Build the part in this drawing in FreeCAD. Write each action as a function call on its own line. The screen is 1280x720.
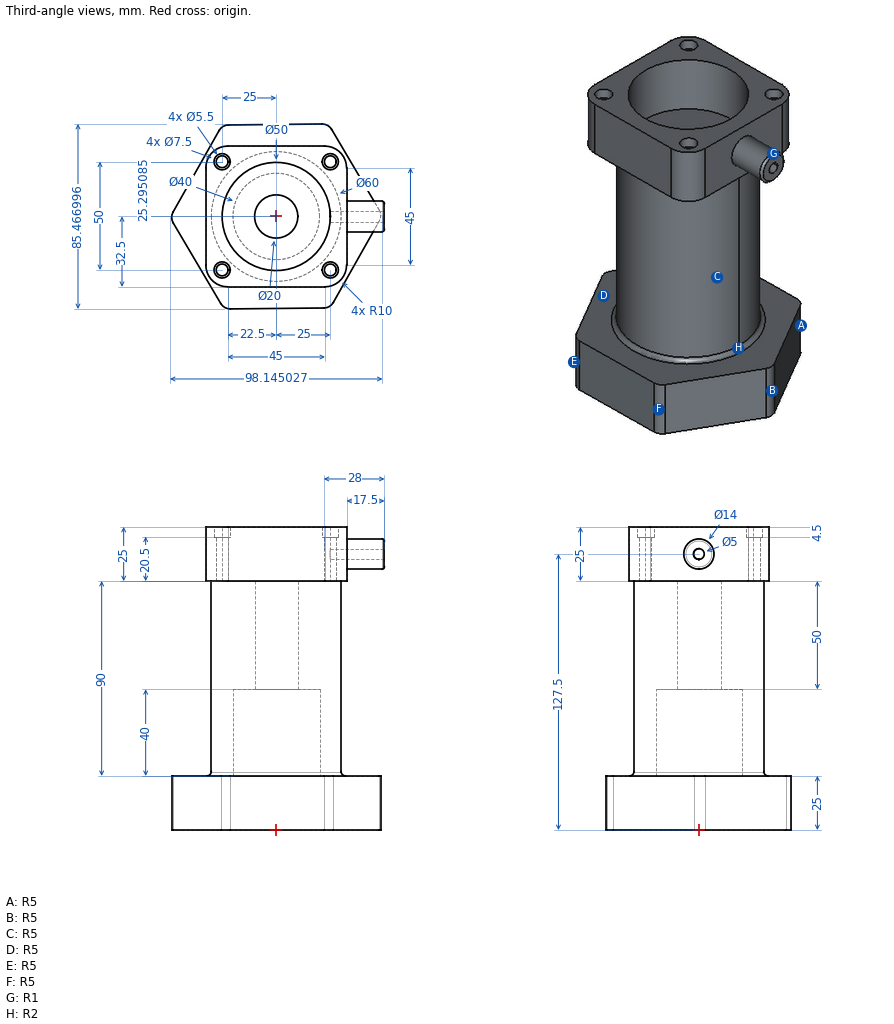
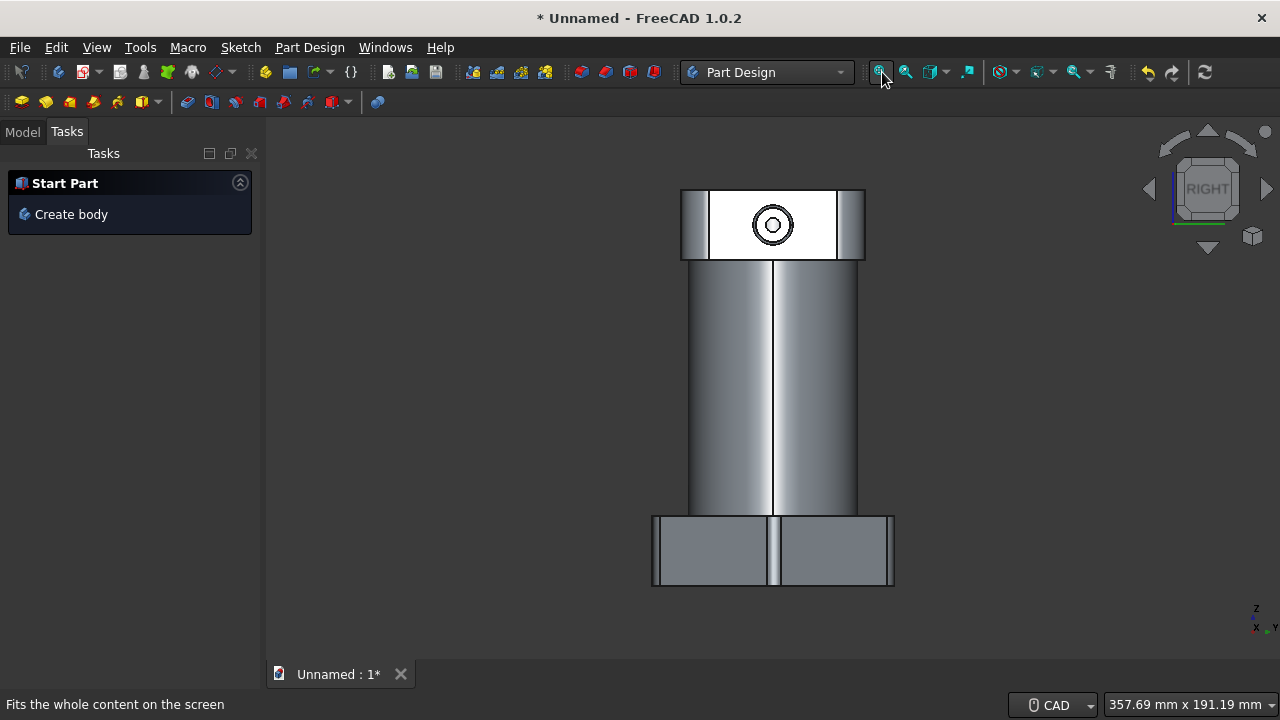
key(5)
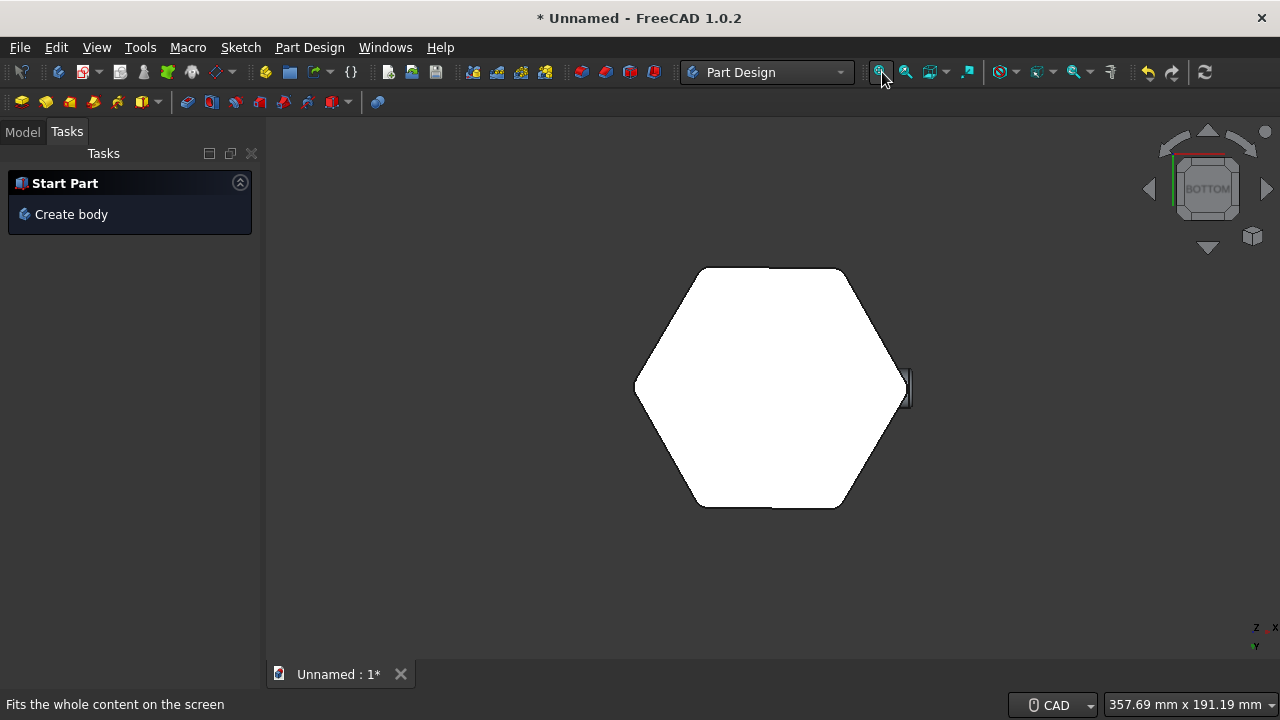
click(882, 72)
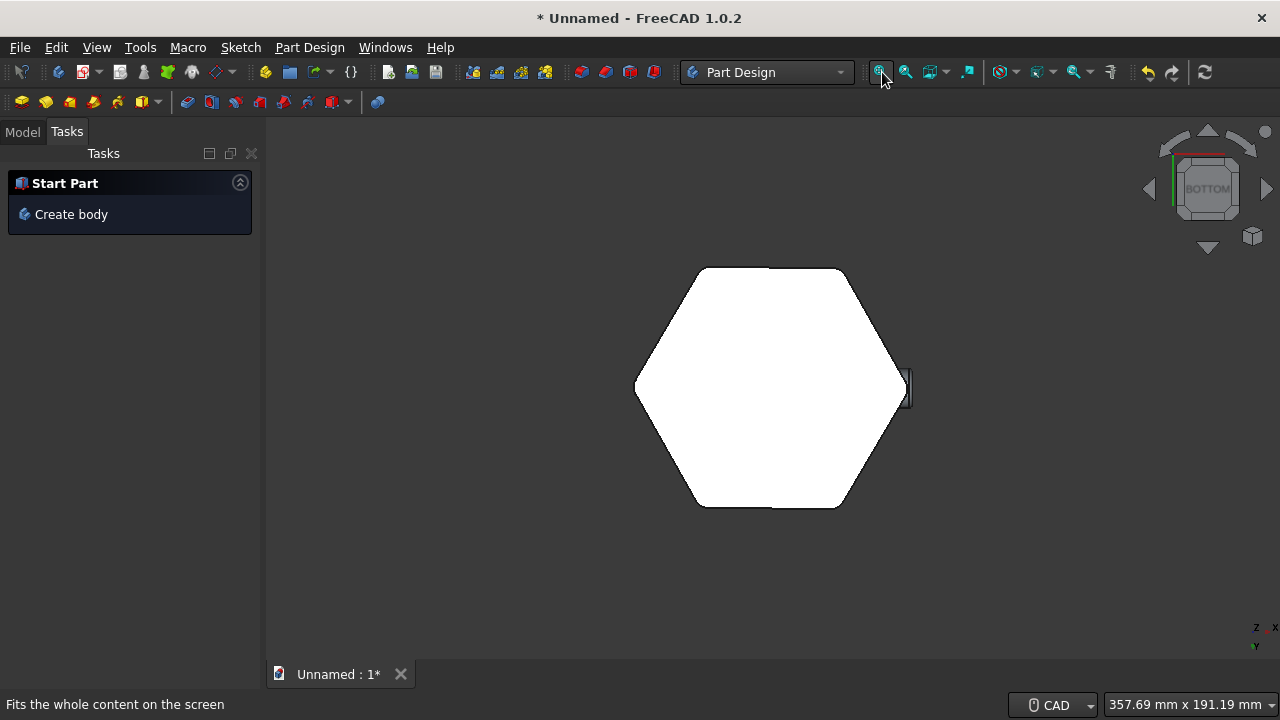
key(4)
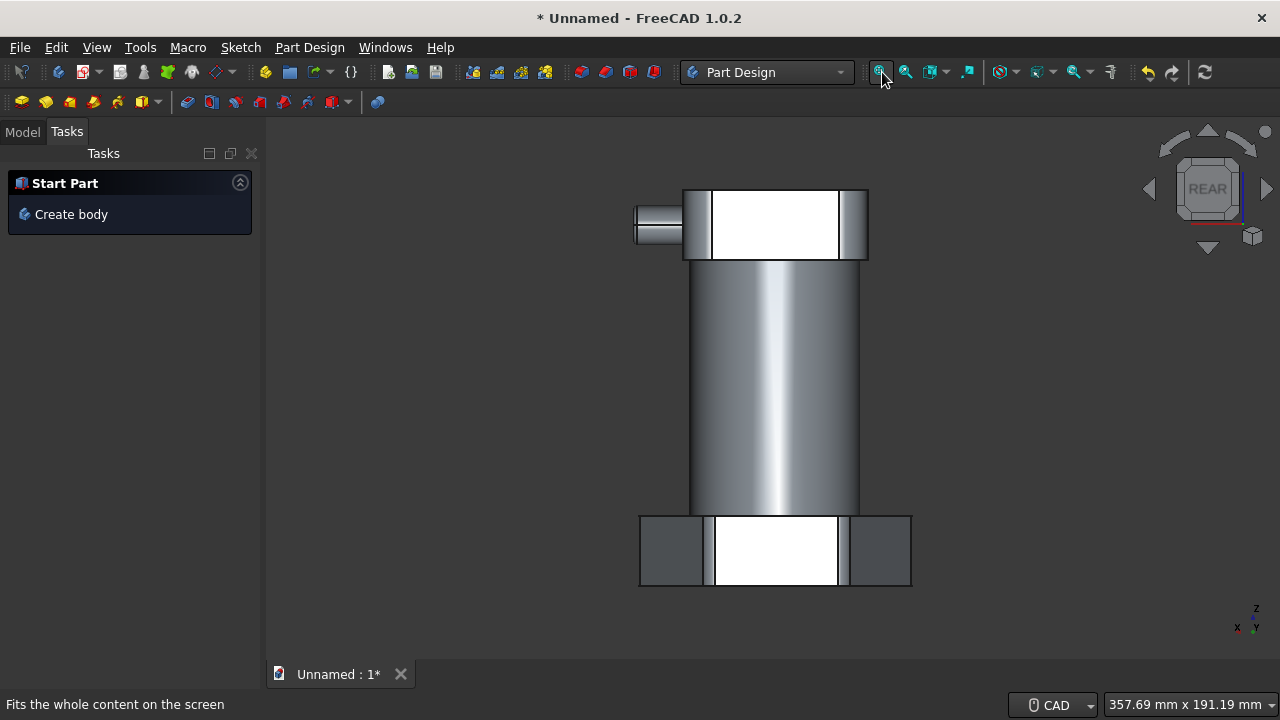
key(6)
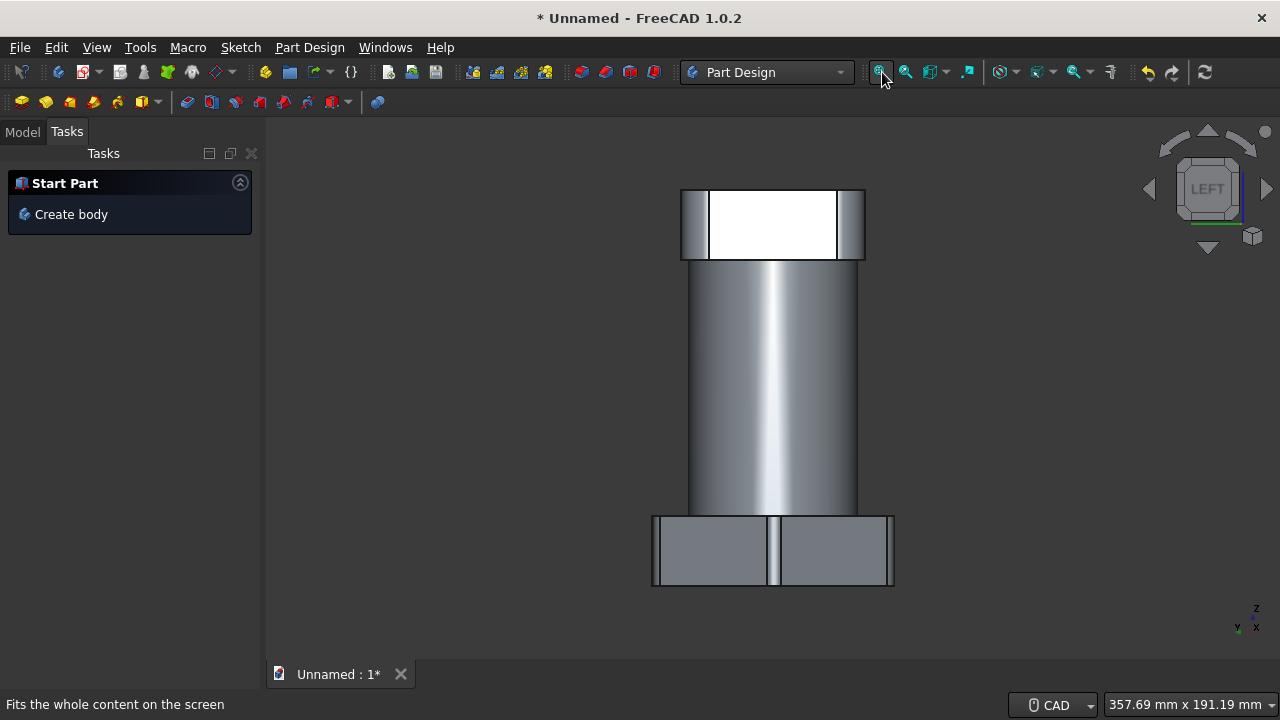
key(v)
key(3)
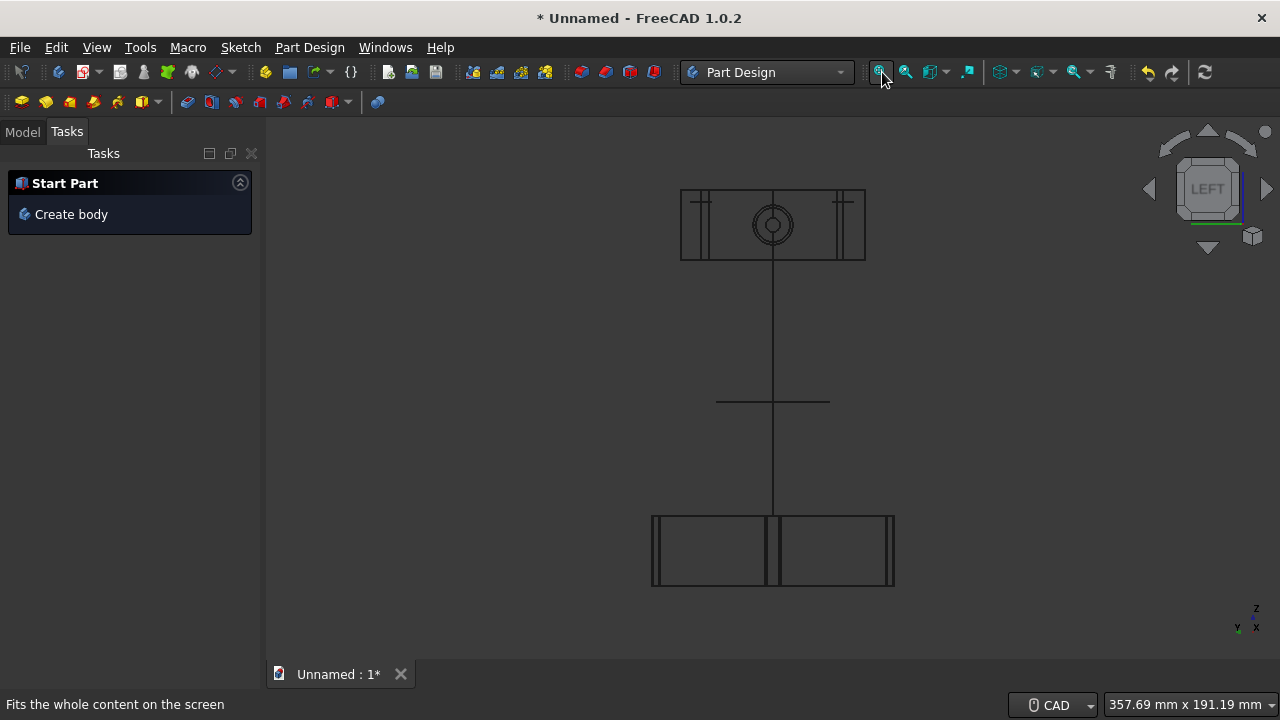
key(0)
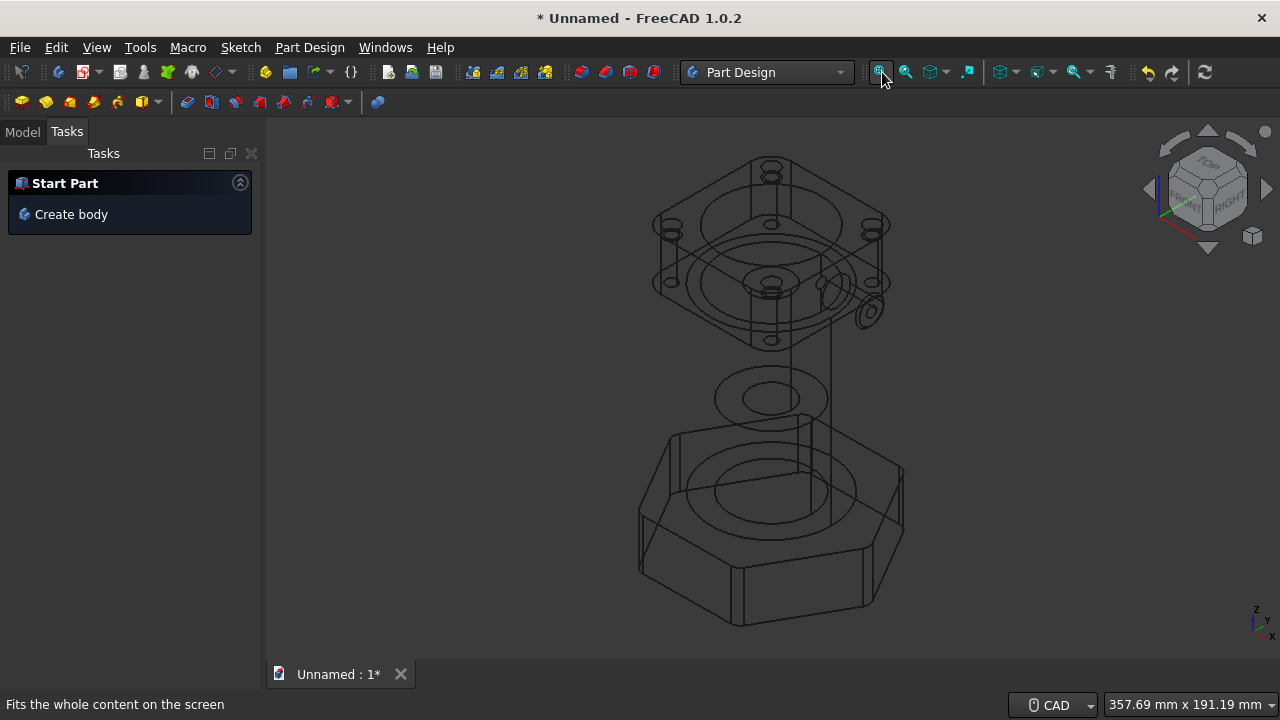
click(711, 455)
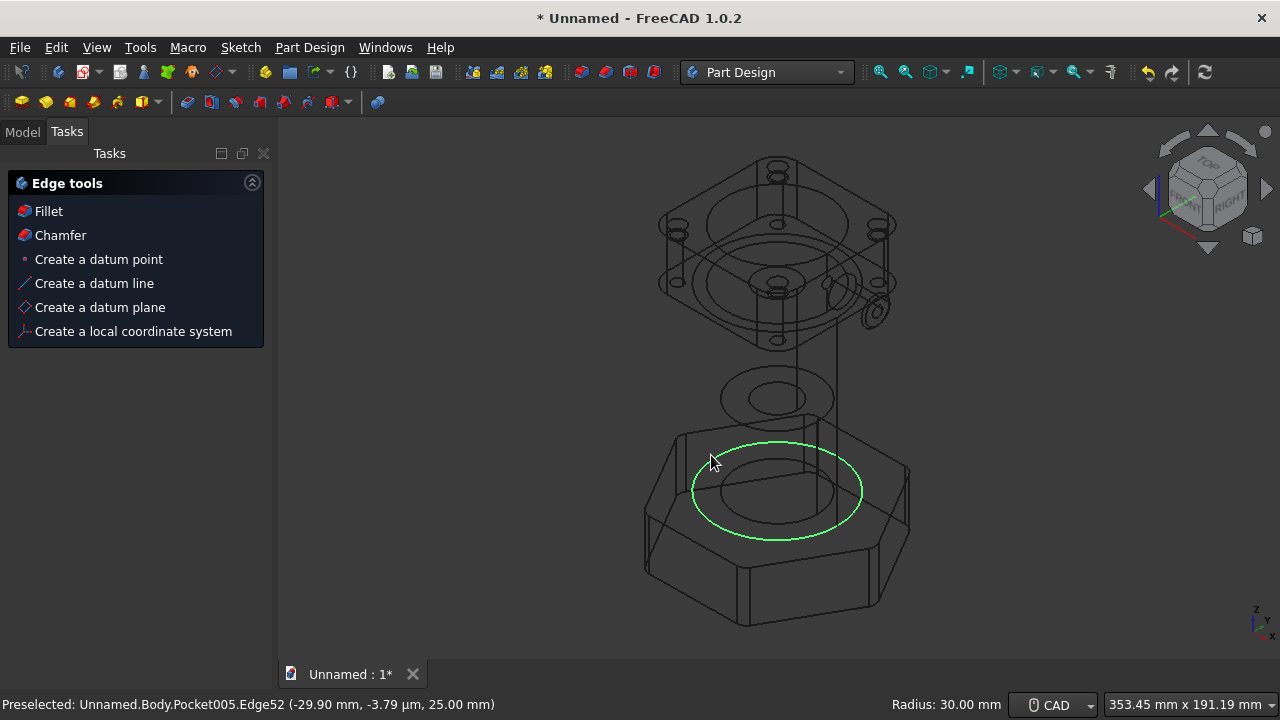
key(v)
key(1)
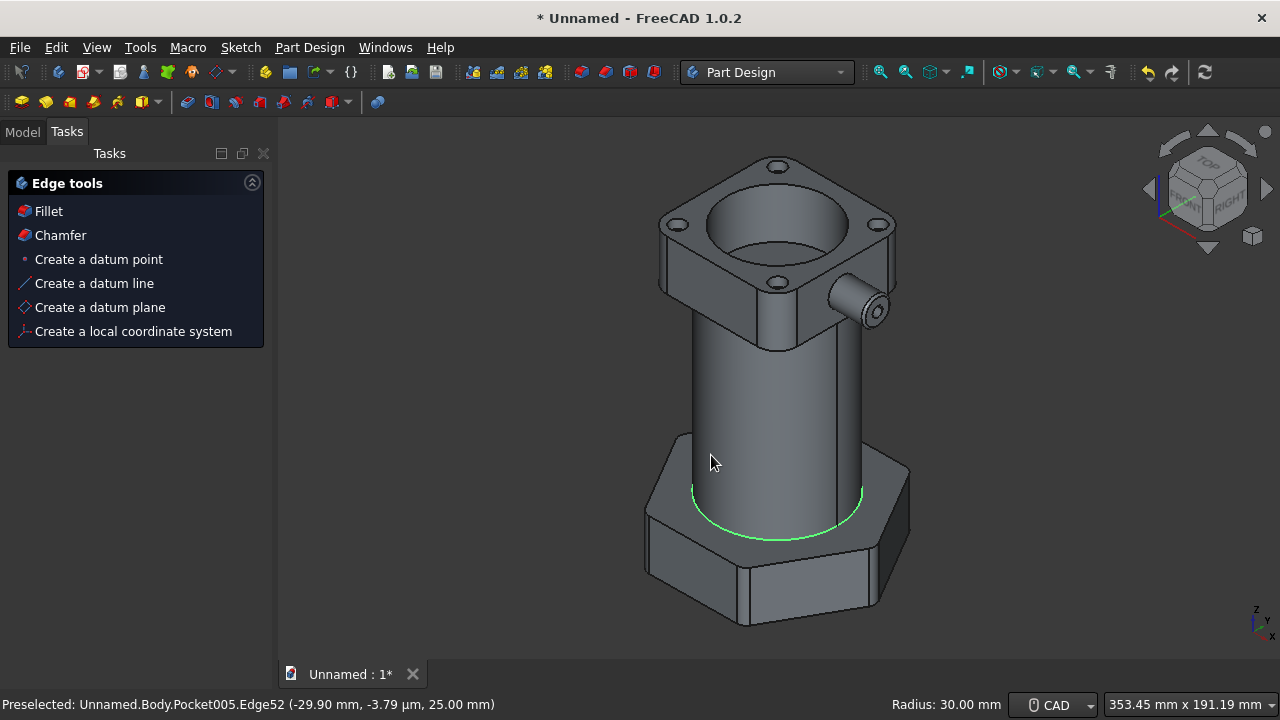
click(582, 72)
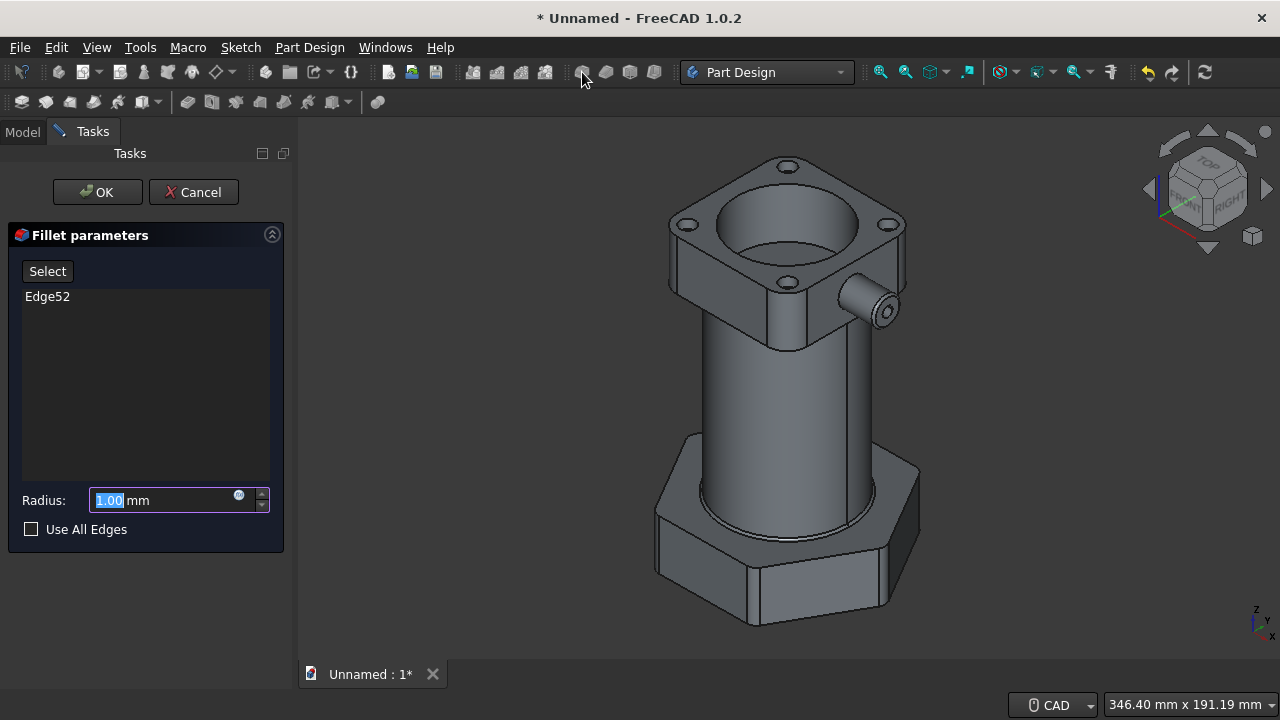
text(2)
key(Tab)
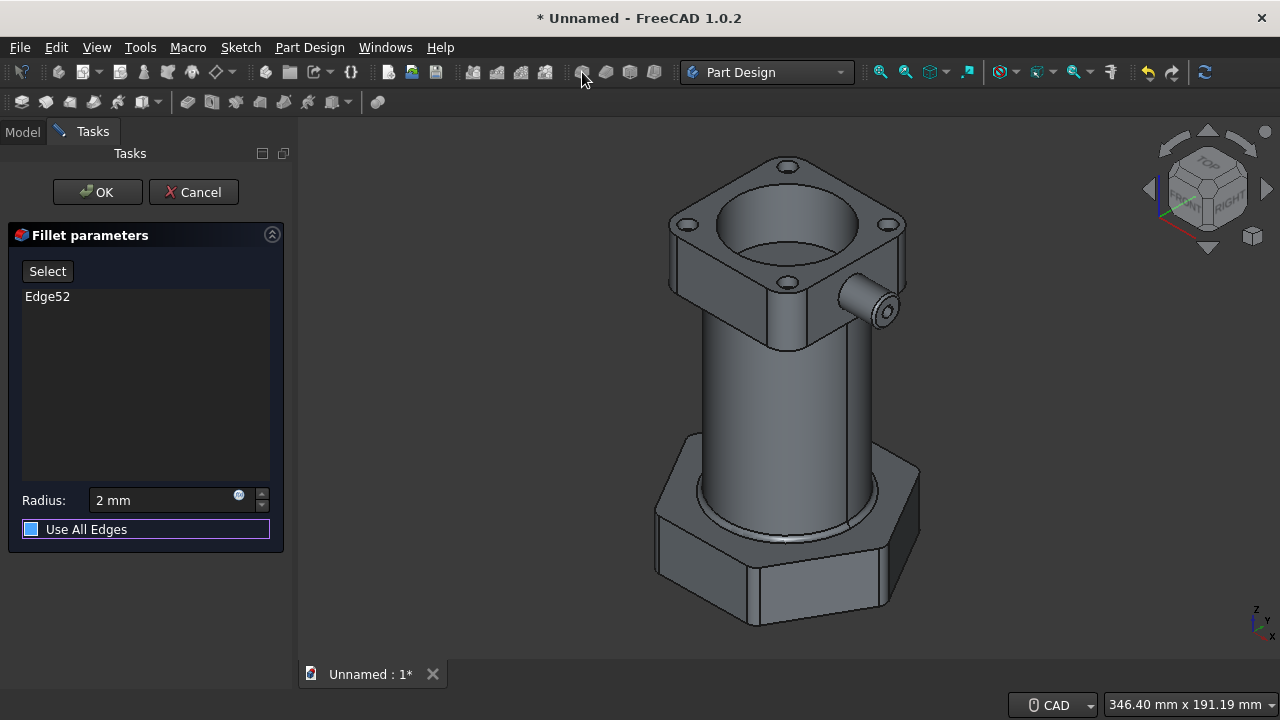
click(98, 192)